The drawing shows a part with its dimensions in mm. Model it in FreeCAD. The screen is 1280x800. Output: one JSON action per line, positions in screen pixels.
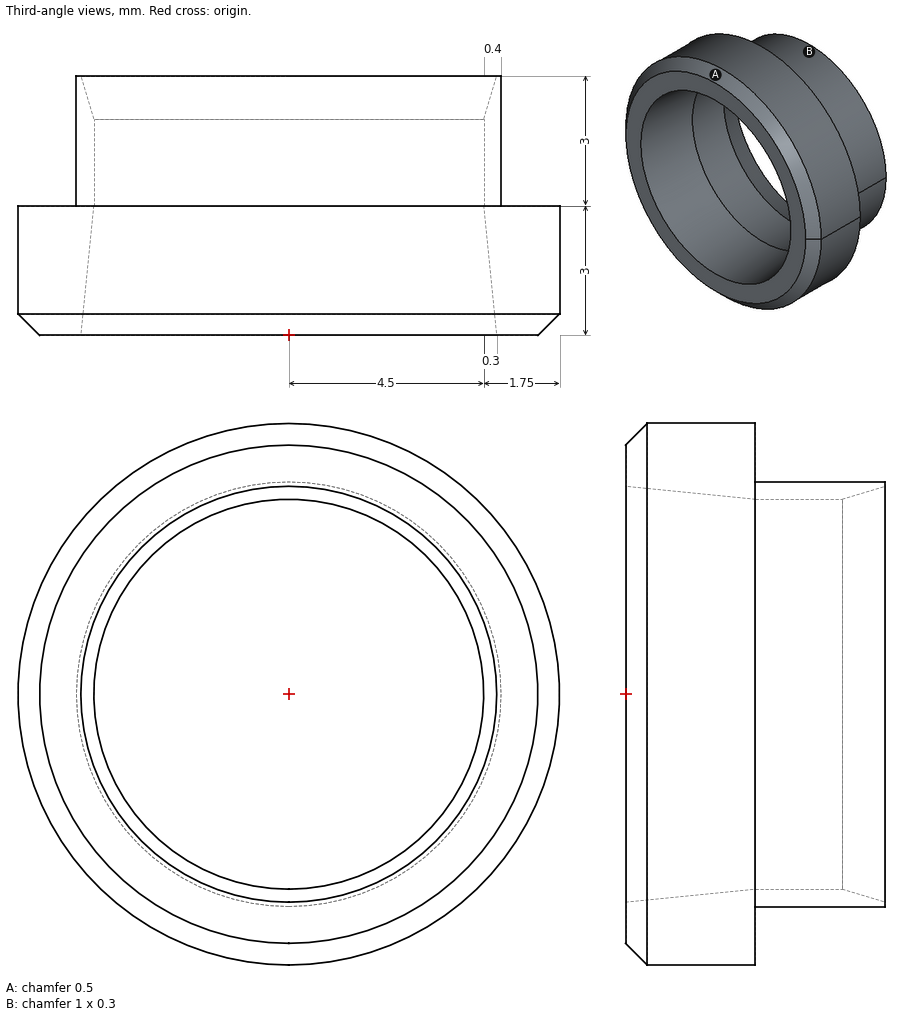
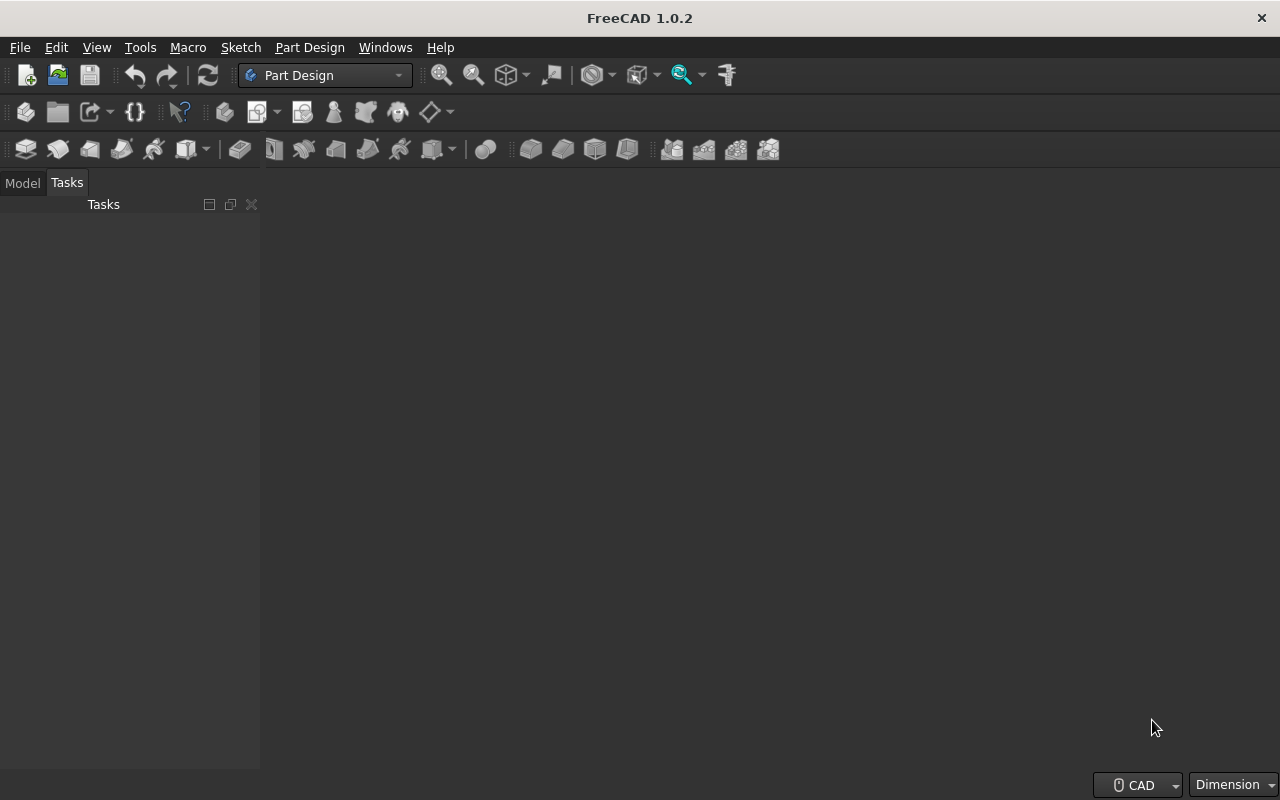
{"action": "left_click", "coordinate": [26, 76]}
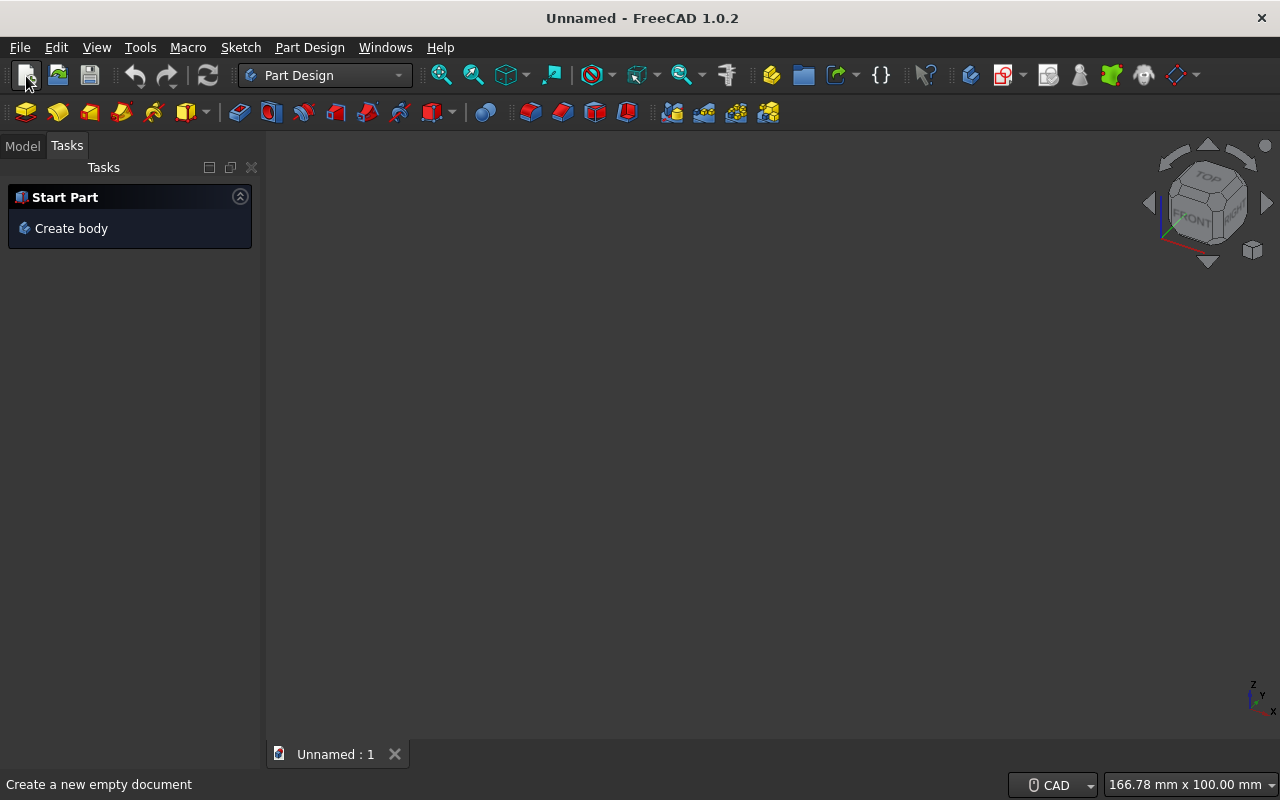
{"action": "left_click", "coordinate": [1004, 76]}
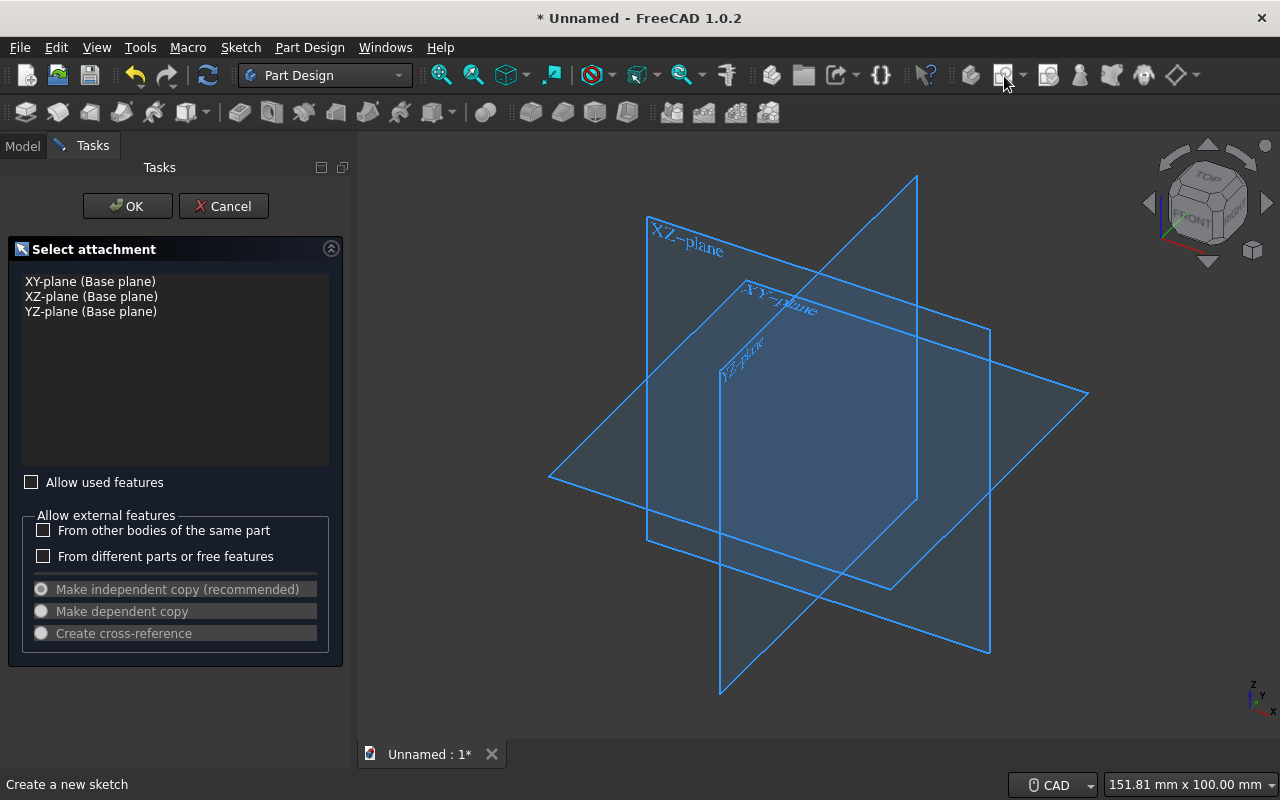
{"action": "left_click", "coordinate": [82, 282]}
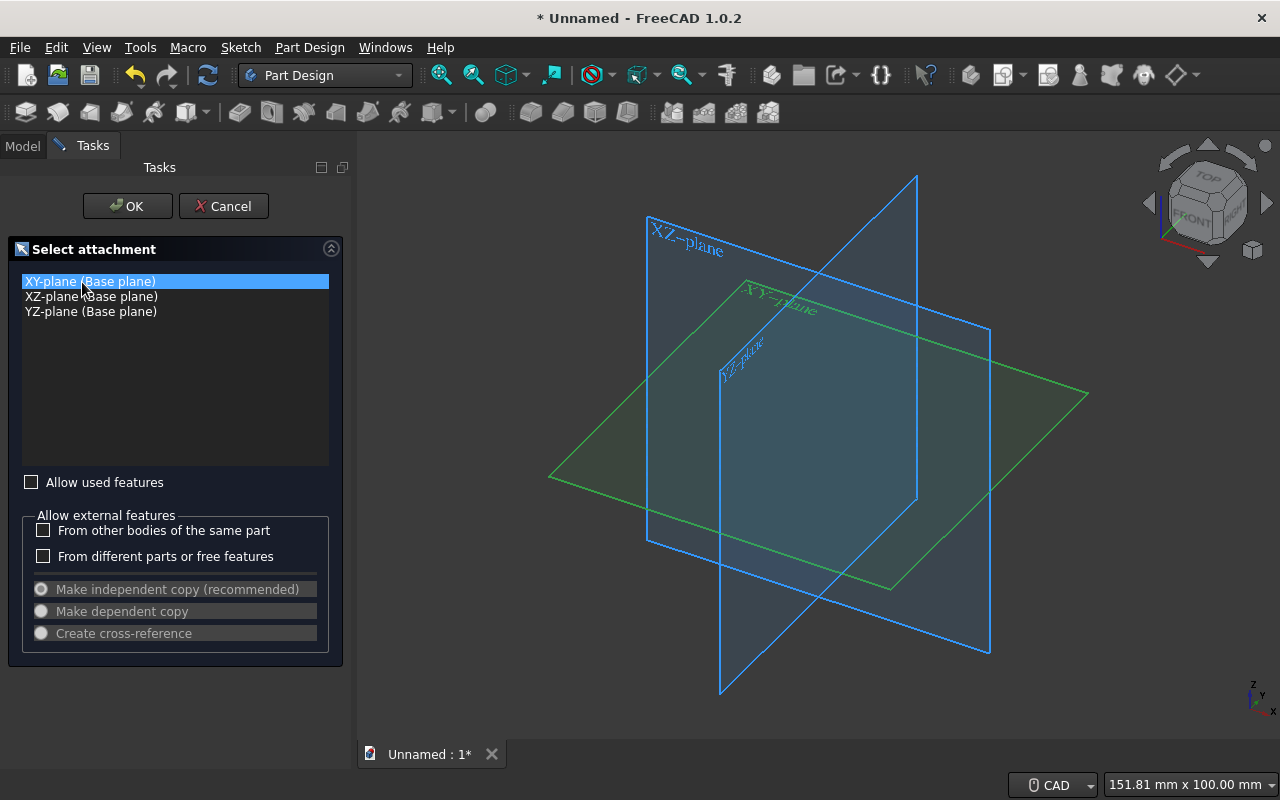
{"action": "left_click", "coordinate": [128, 206]}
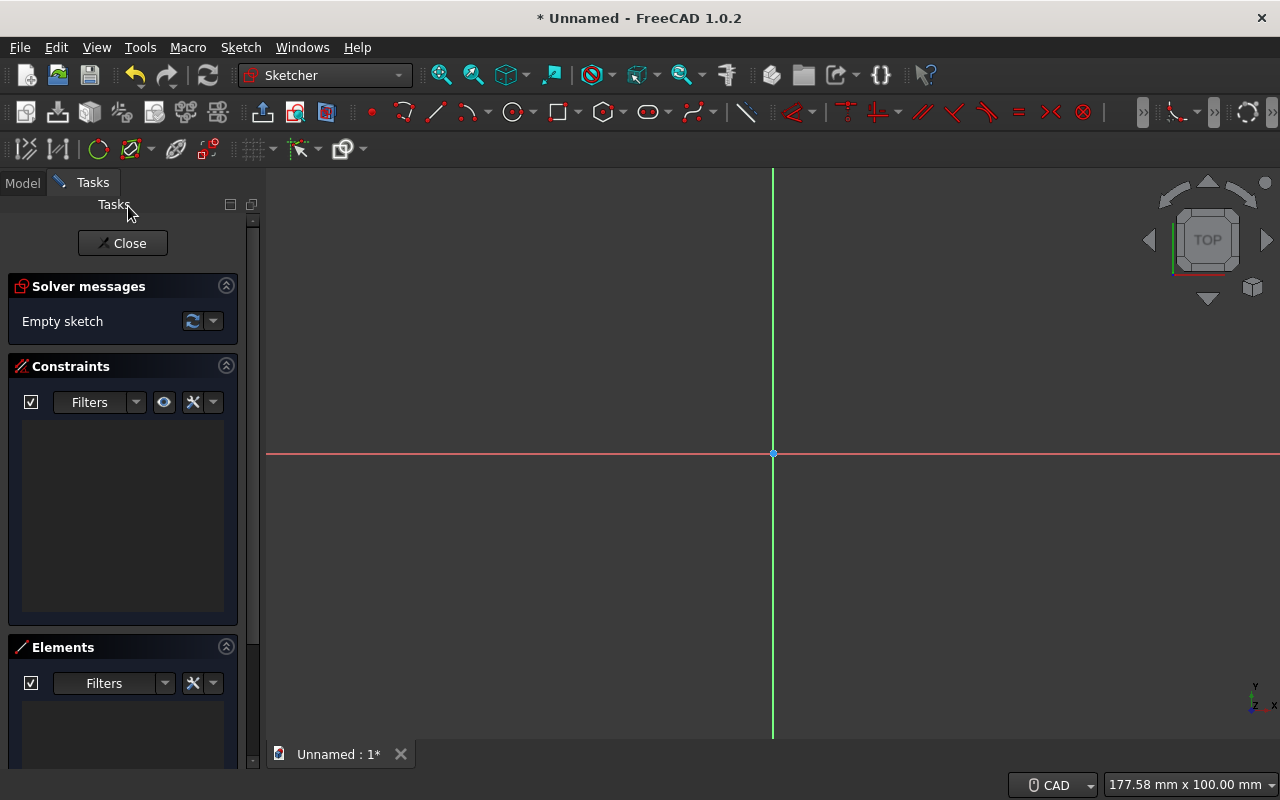
{"action": "scroll", "coordinate": [799, 435], "scroll_direction": "up", "scroll_amount": 12}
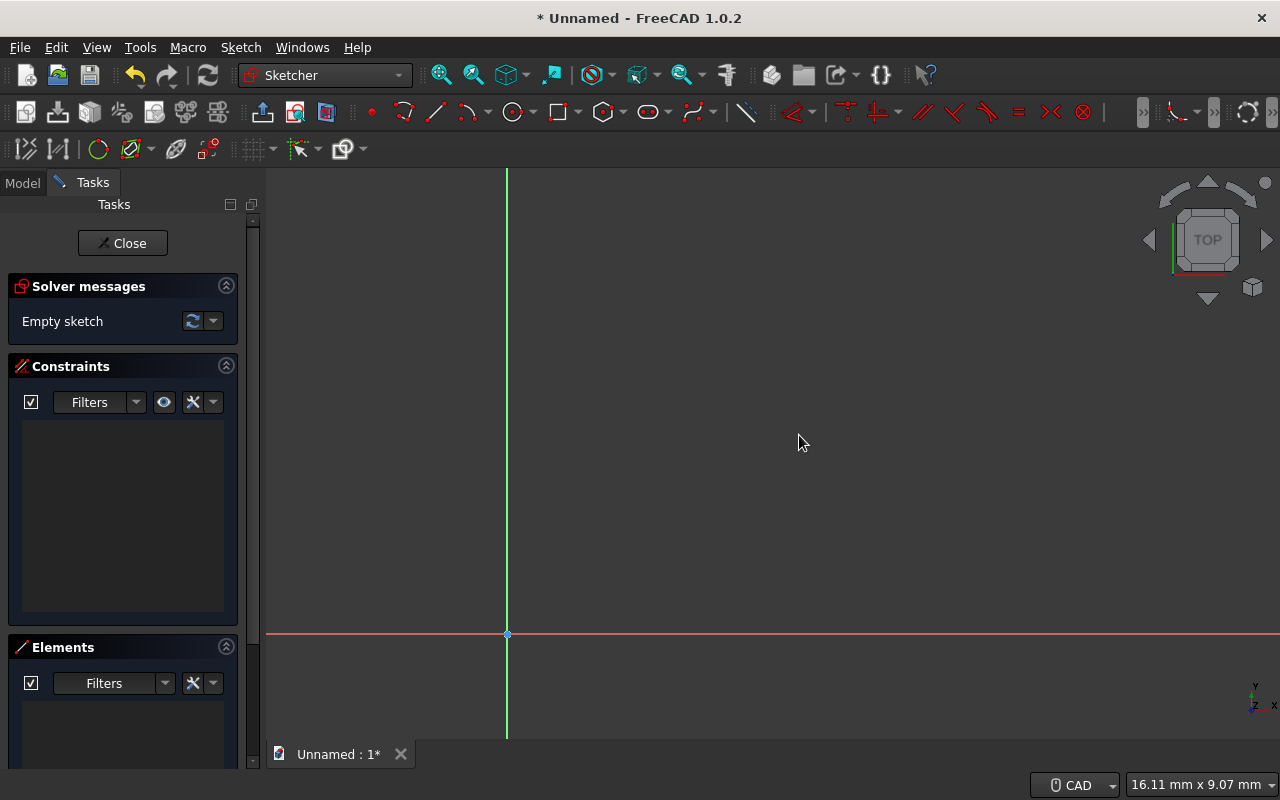
{"action": "key", "text": "g m"}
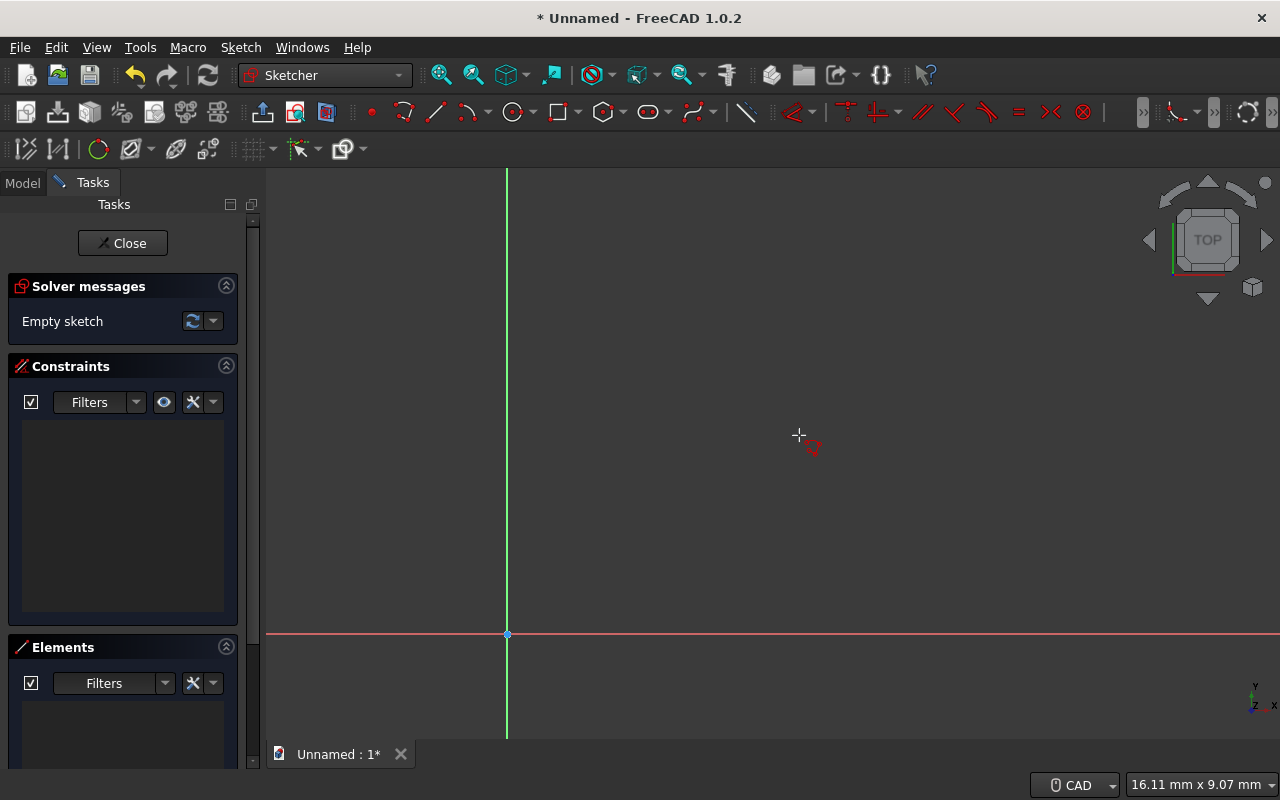
{"action": "left_click", "coordinate": [790, 634]}
{"action": "left_click", "coordinate": [901, 625]}
{"action": "left_click", "coordinate": [901, 445]}
{"action": "left_click", "coordinate": [816, 445]}
{"action": "left_click", "coordinate": [816, 257]}
{"action": "left_click", "coordinate": [790, 257]}
{"action": "left_click", "coordinate": [790, 634]}
{"action": "key", "text": "Escape"}
{"action": "key", "text": "Escape"}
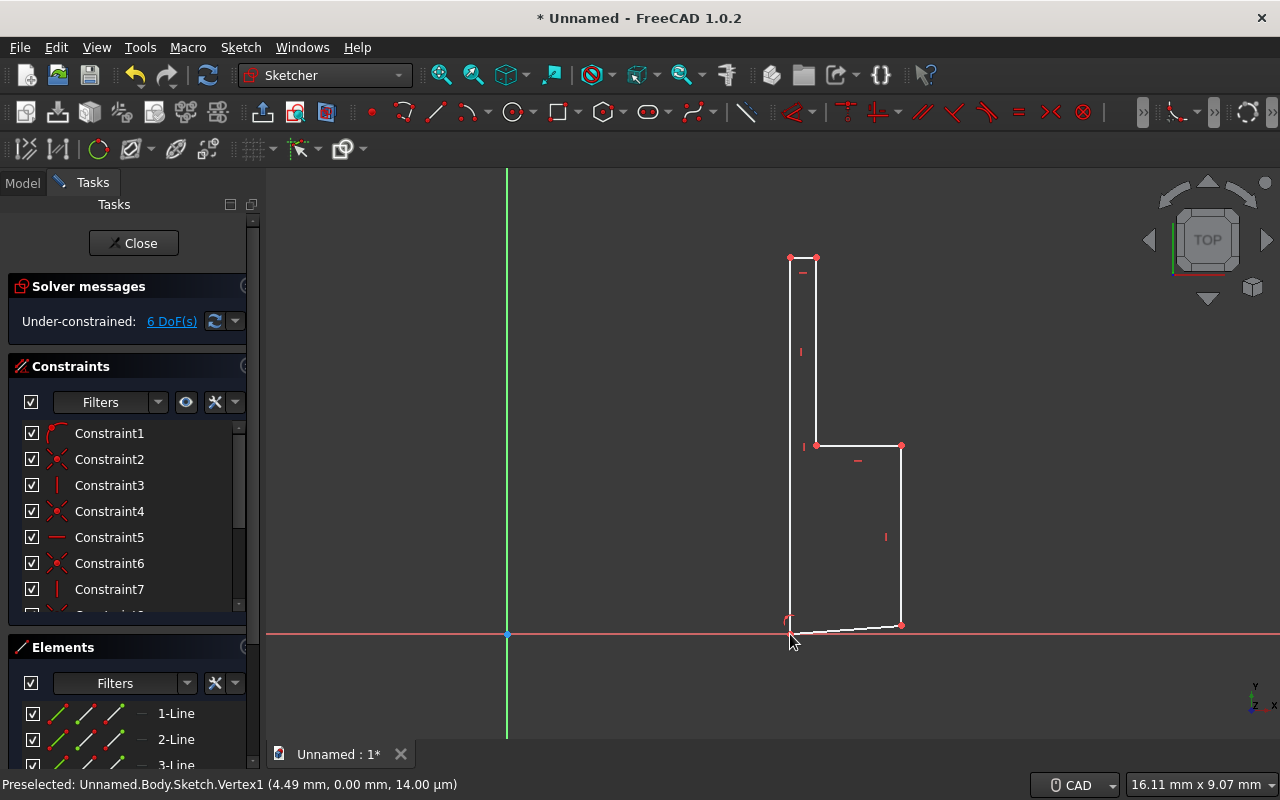
{"action": "left_click", "coordinate": [823, 632]}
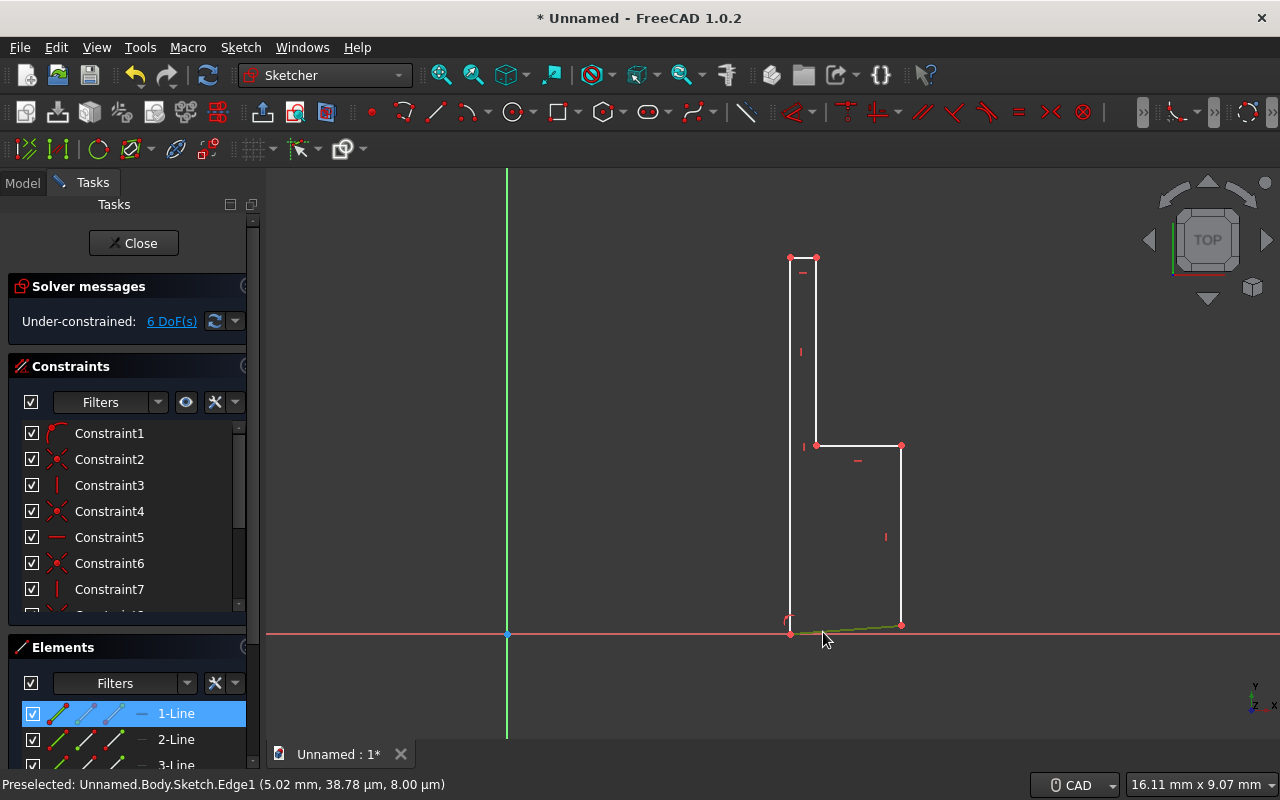
{"action": "left_click", "coordinate": [900, 112]}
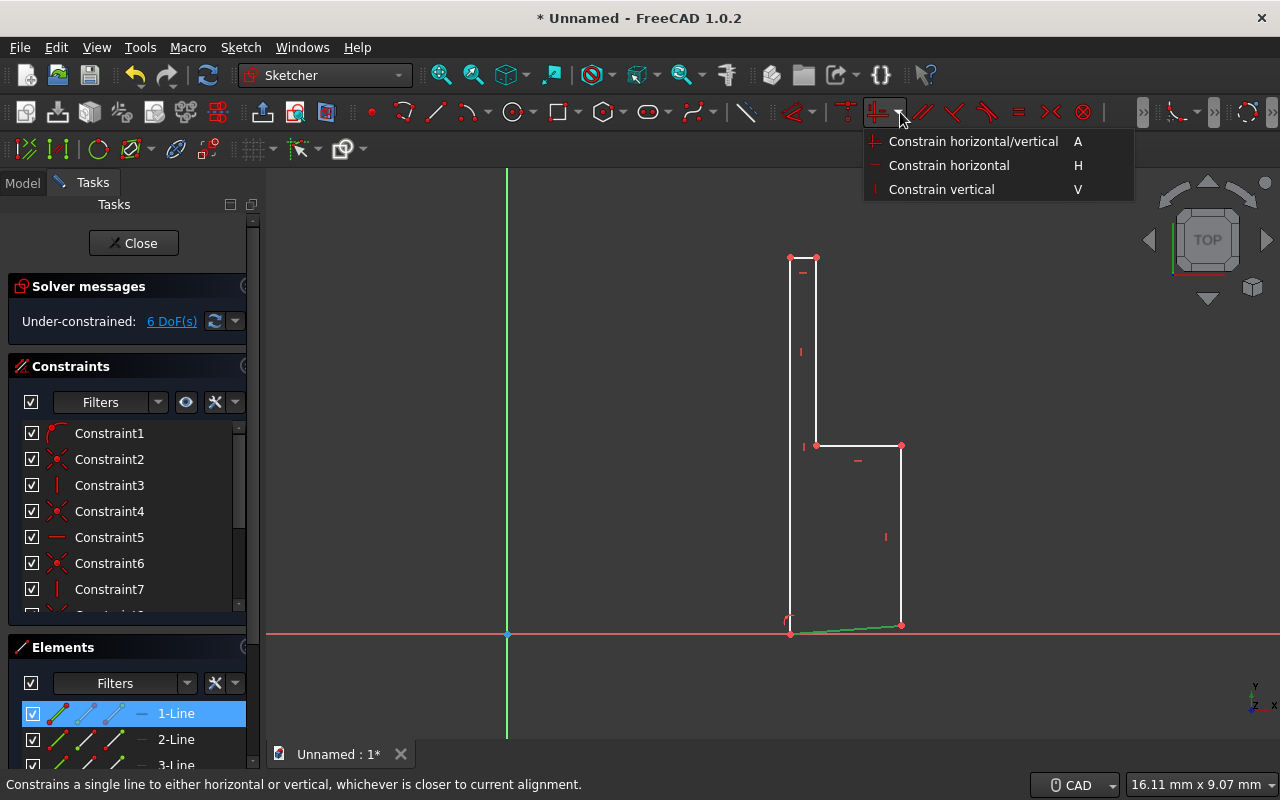
{"action": "left_click", "coordinate": [999, 165]}